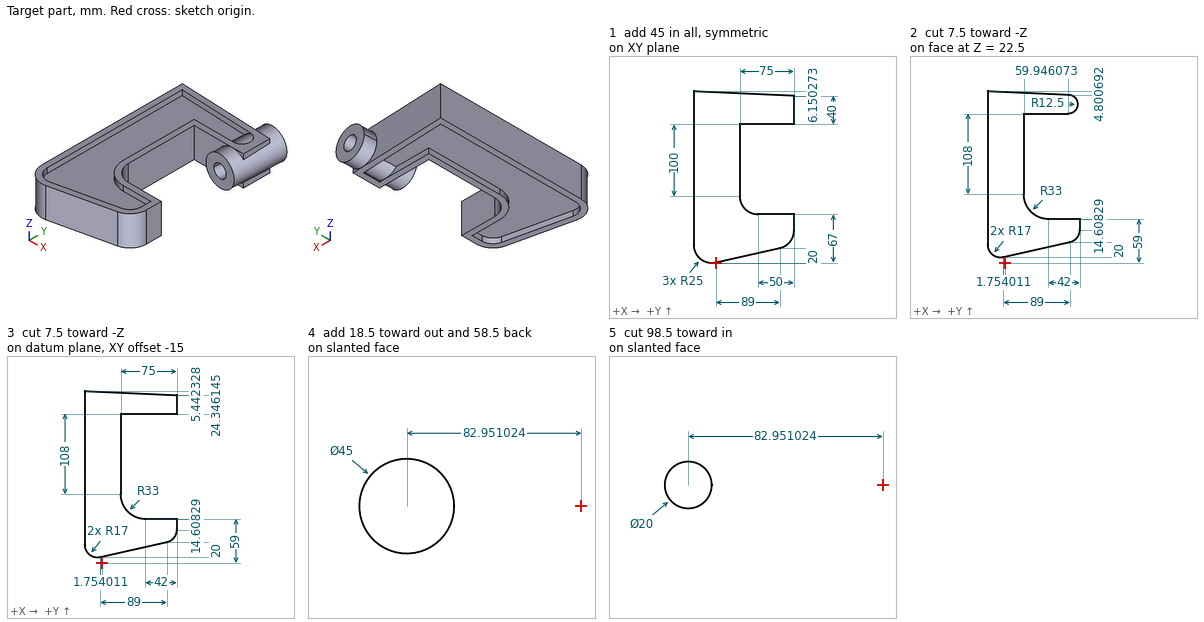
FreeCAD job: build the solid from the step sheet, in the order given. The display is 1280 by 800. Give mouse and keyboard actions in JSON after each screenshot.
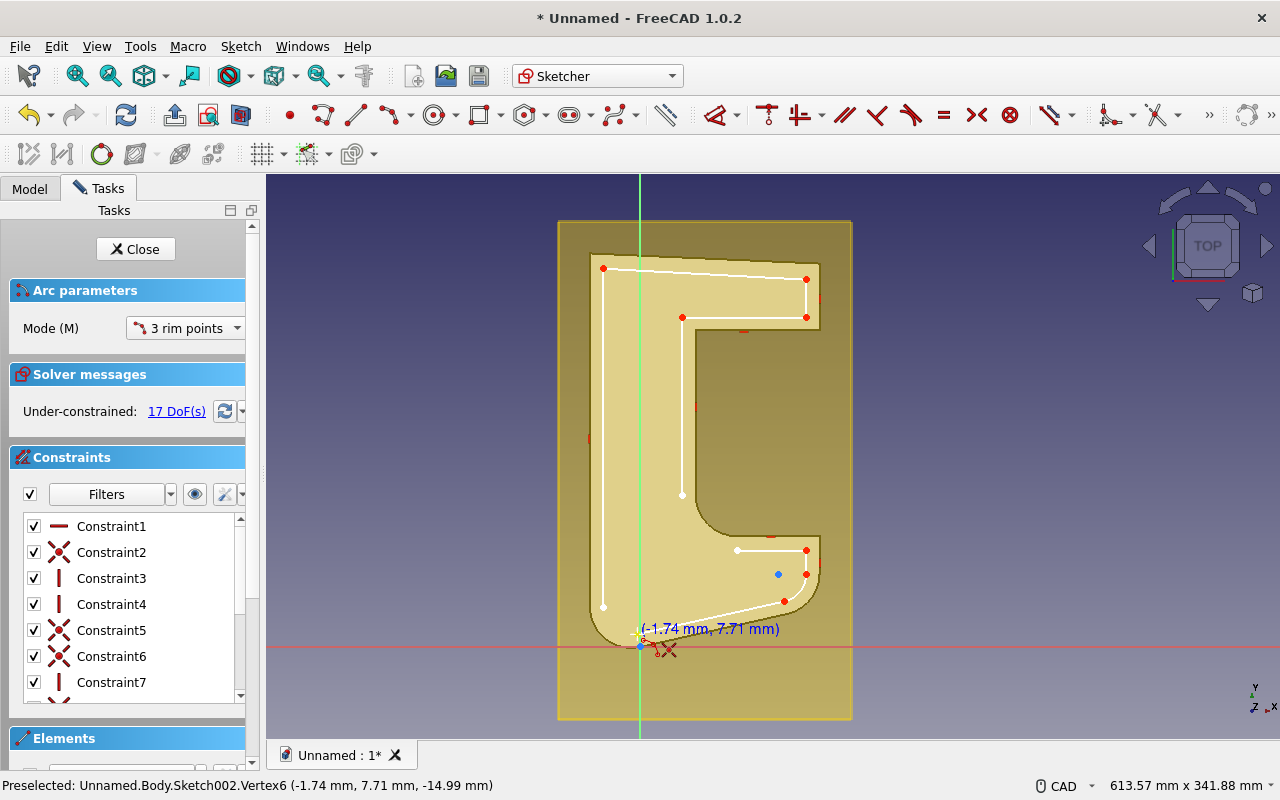
{"action": "left_click", "coordinate": [603, 608]}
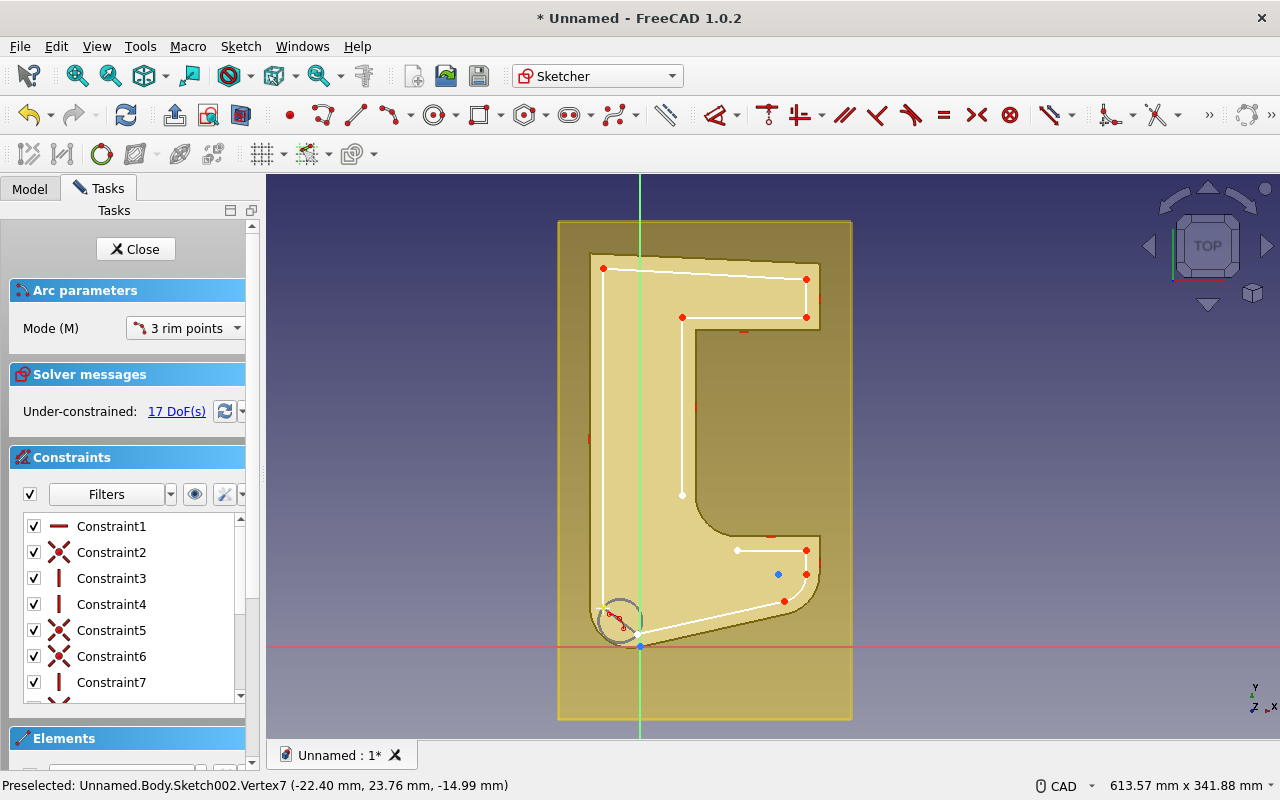
{"action": "scroll", "coordinate": [614, 629], "scroll_direction": "up", "scroll_amount": 3}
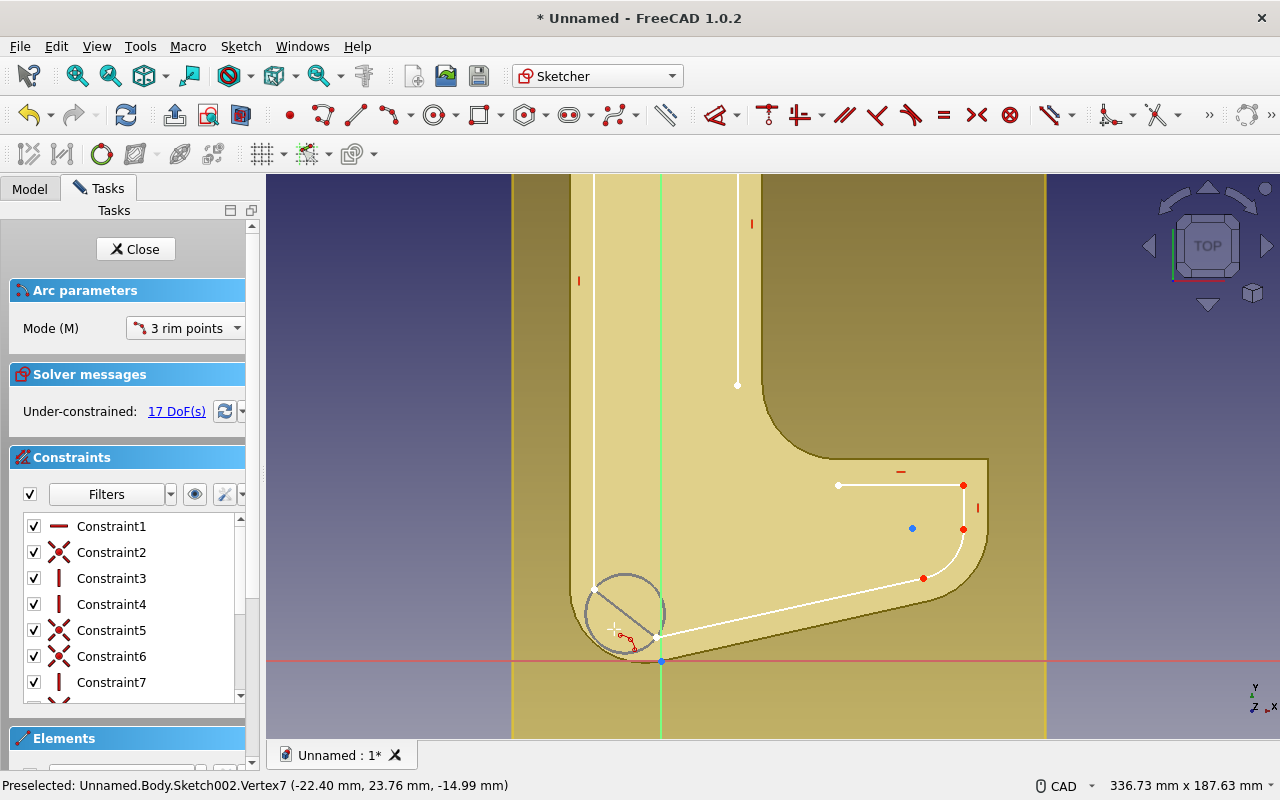
{"action": "left_click", "coordinate": [613, 628]}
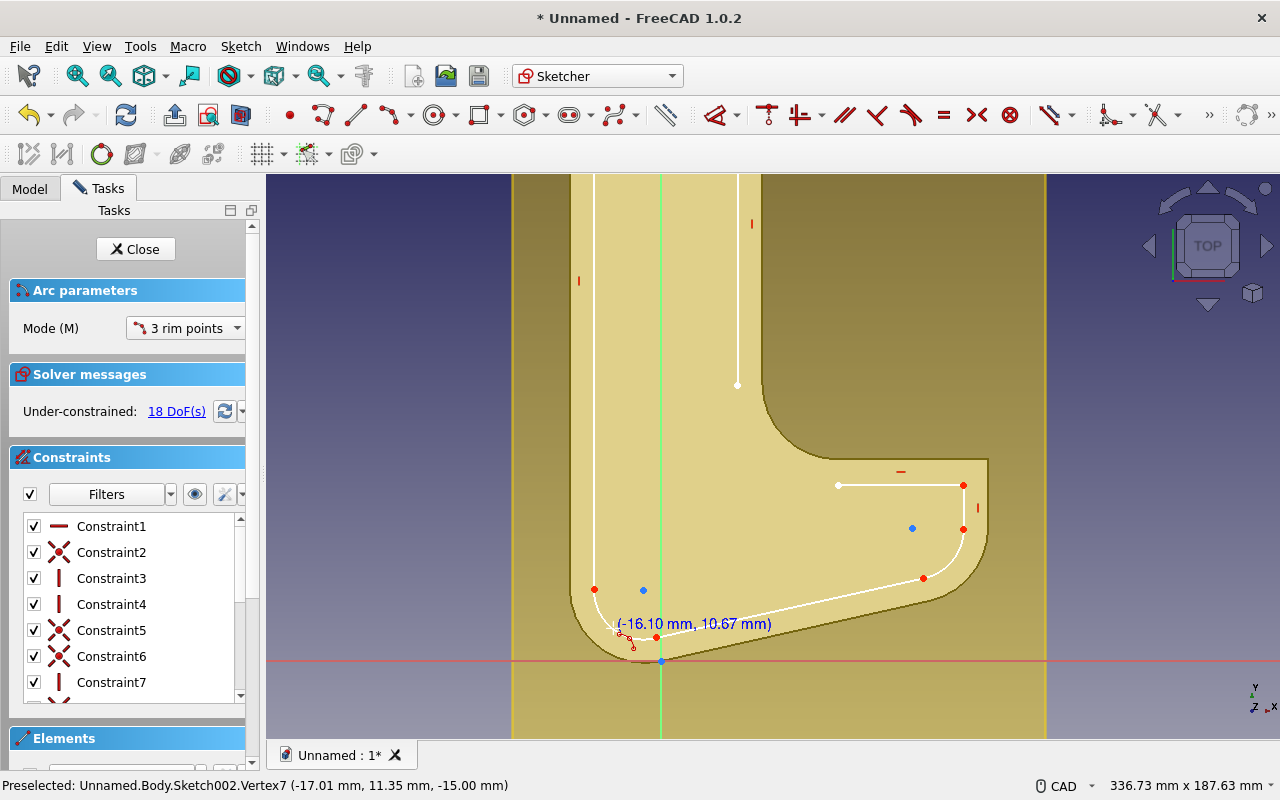
{"action": "left_click", "coordinate": [738, 385]}
{"action": "left_click", "coordinate": [838, 485]}
{"action": "left_click", "coordinate": [767, 454]}
{"action": "key", "text": "Escape"}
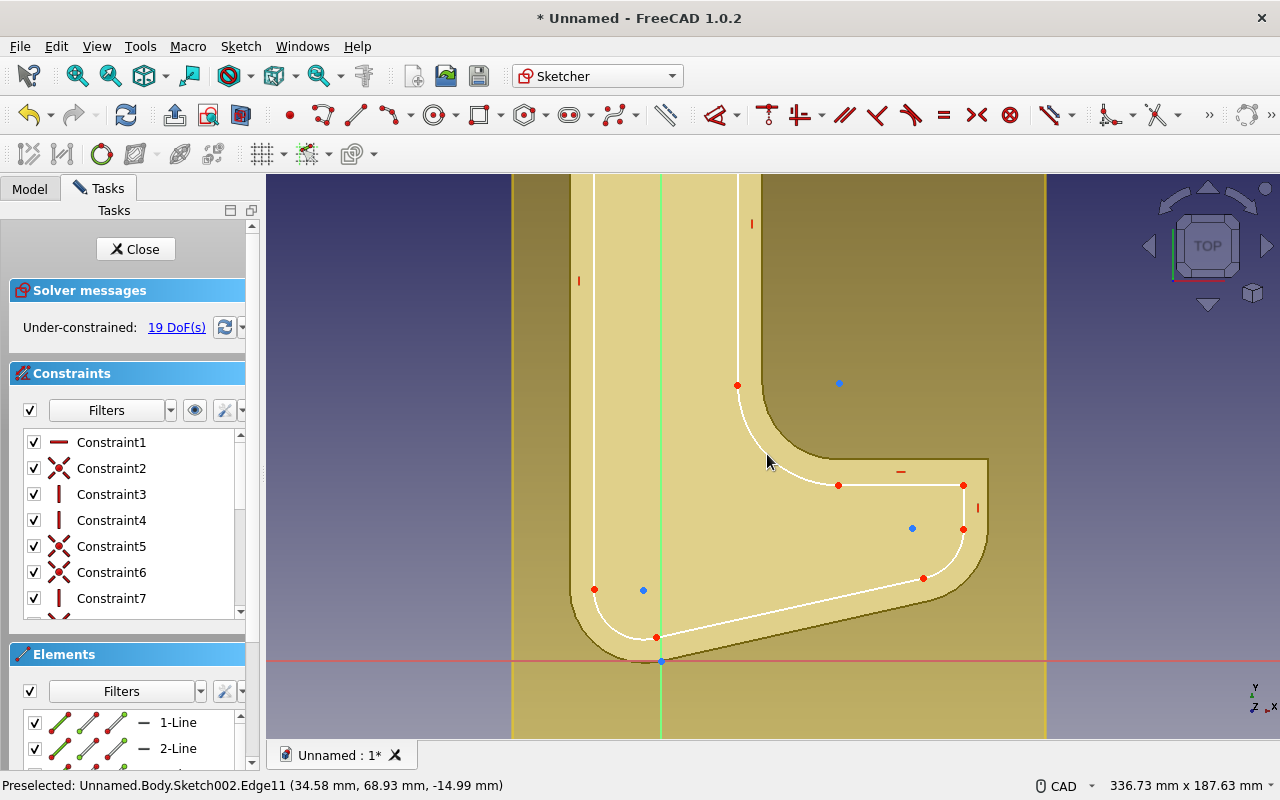
{"action": "left_click", "coordinate": [876, 485]}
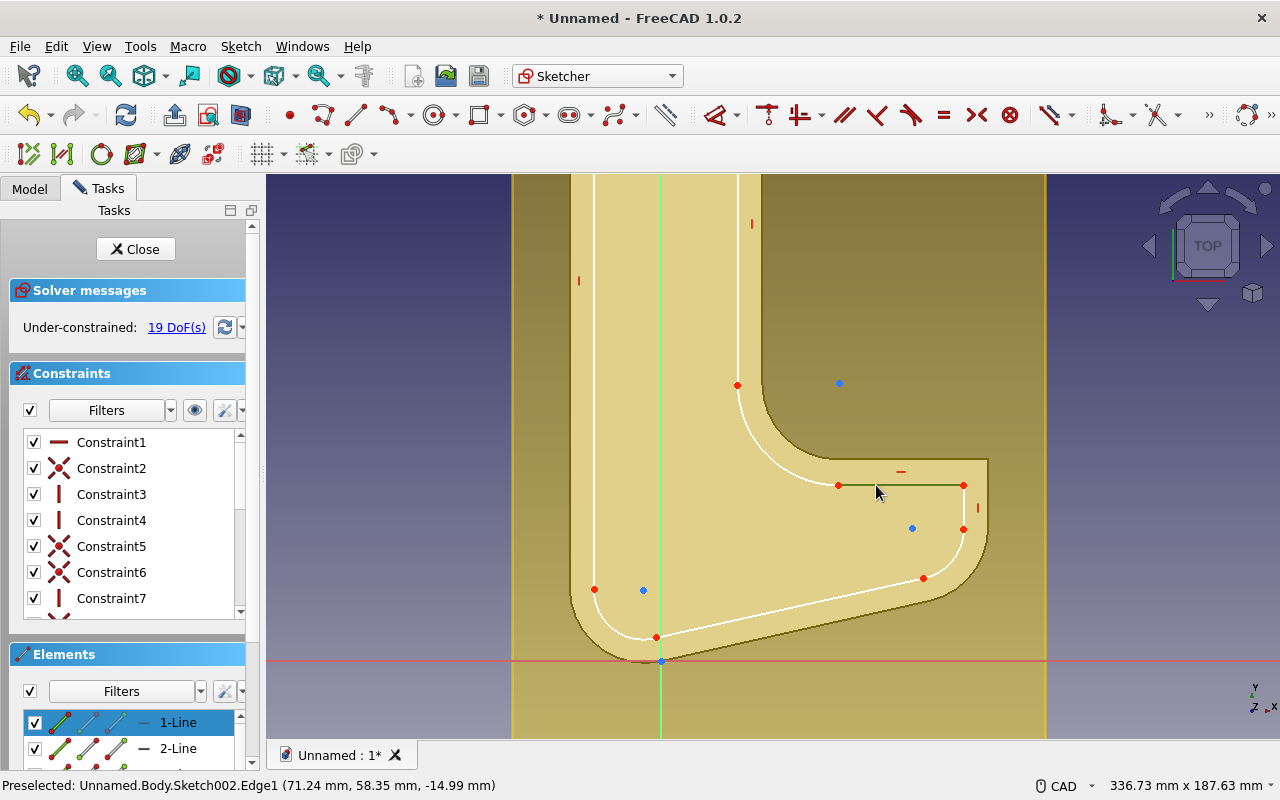
{"action": "left_click", "coordinate": [749, 431]}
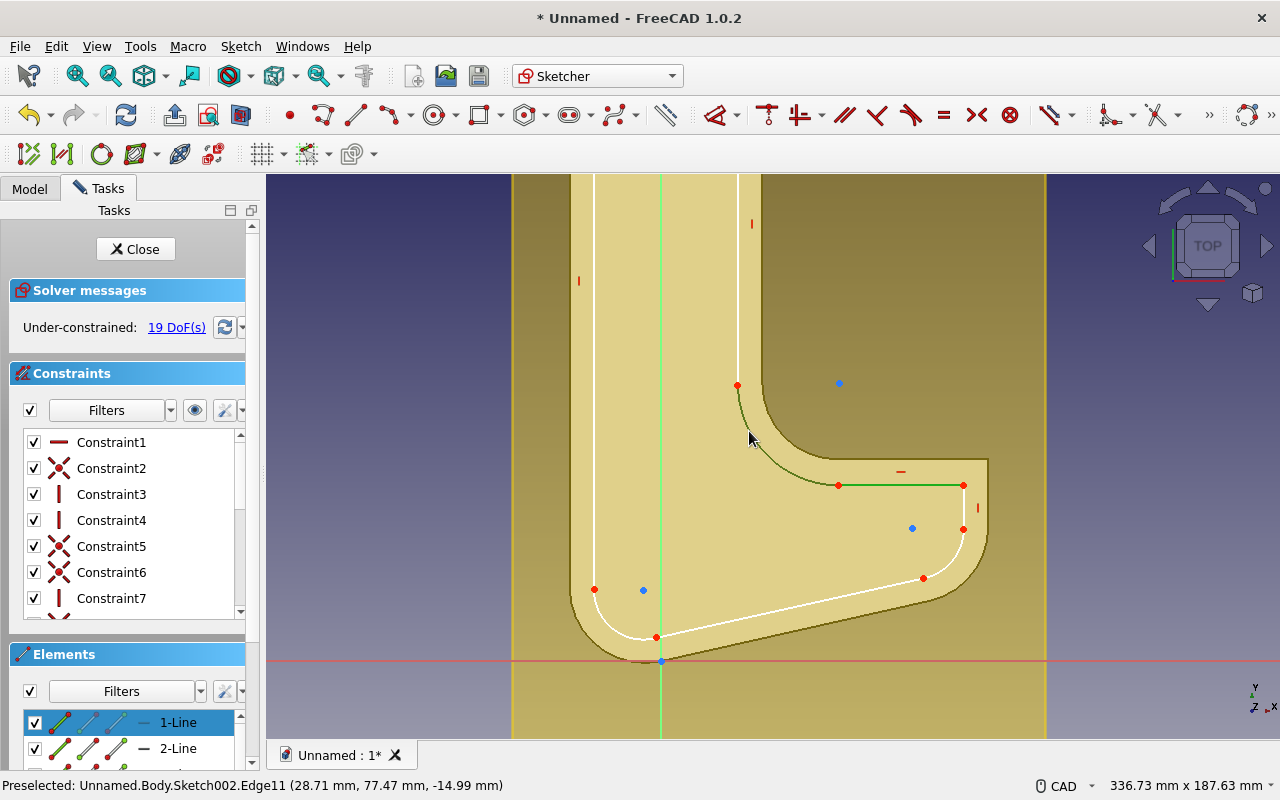
{"action": "left_click", "coordinate": [911, 116]}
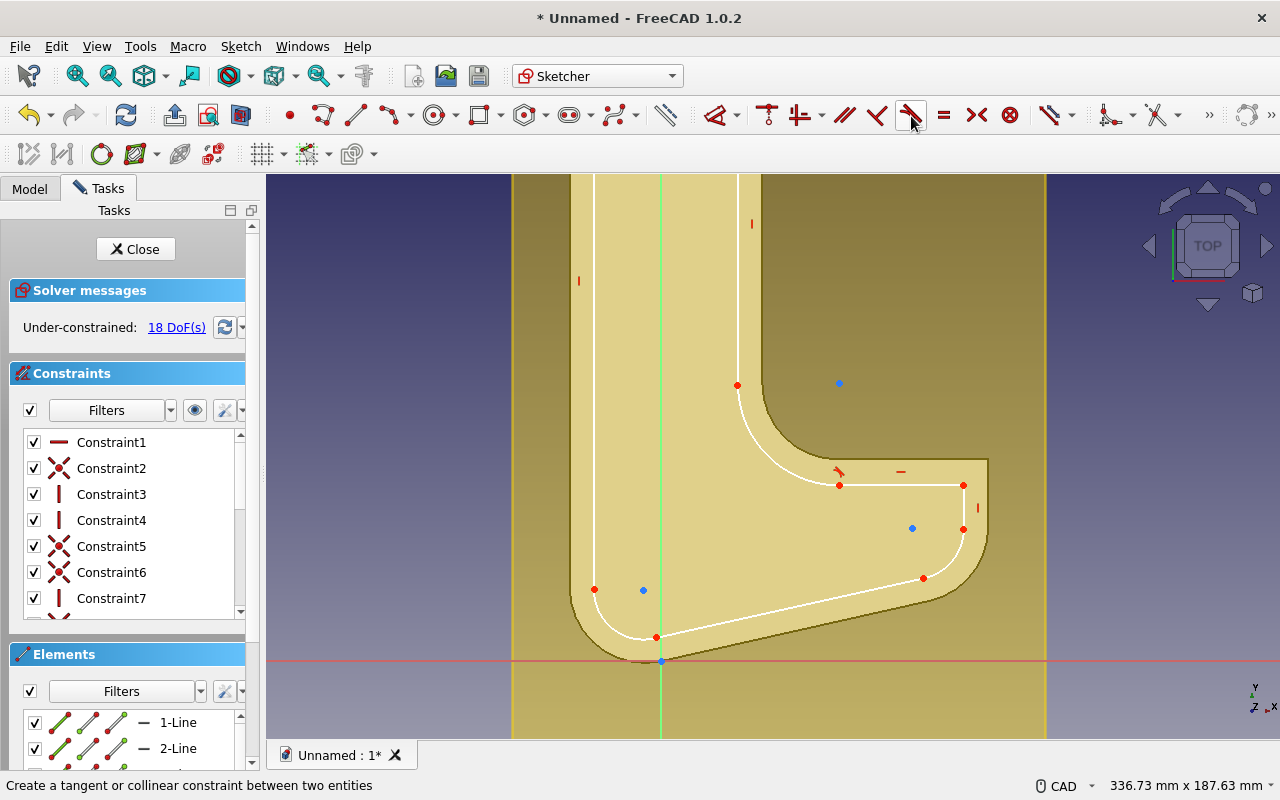
{"action": "left_click", "coordinate": [964, 499]}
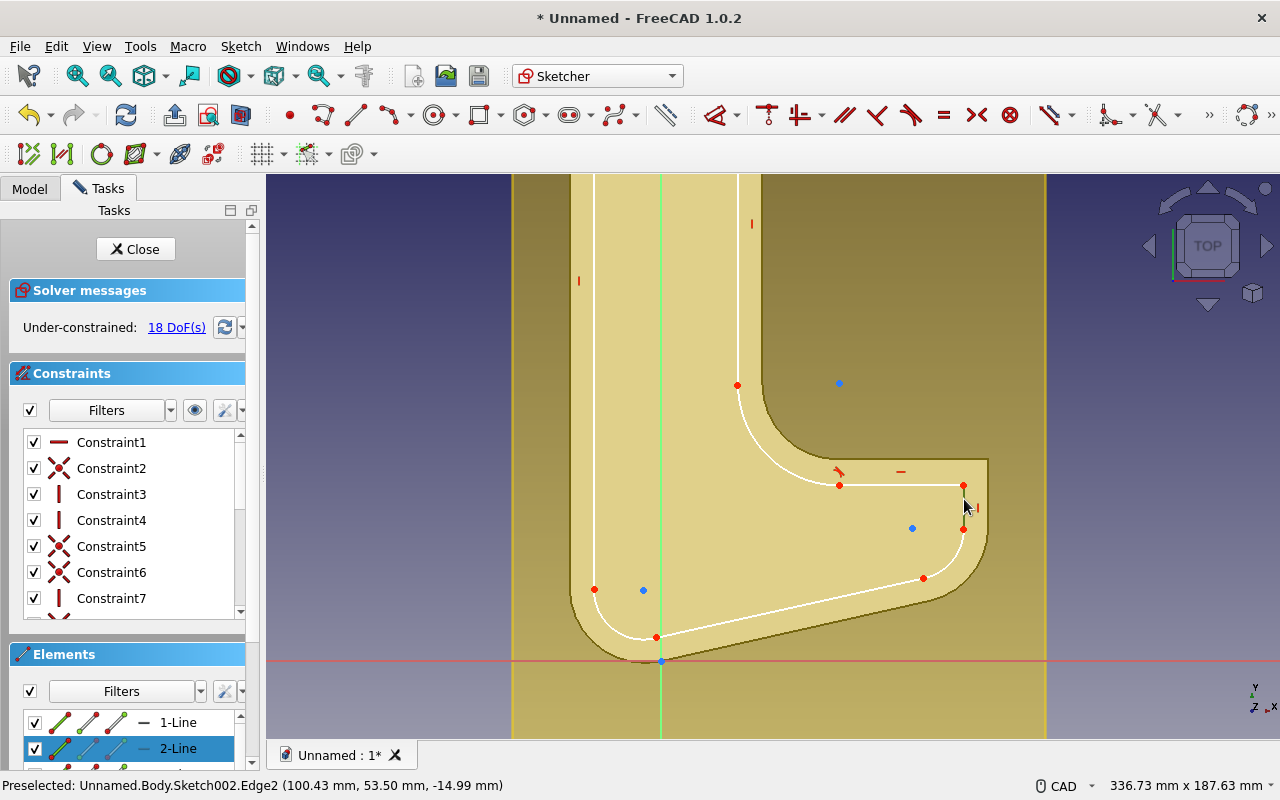
{"action": "left_click", "coordinate": [942, 570]}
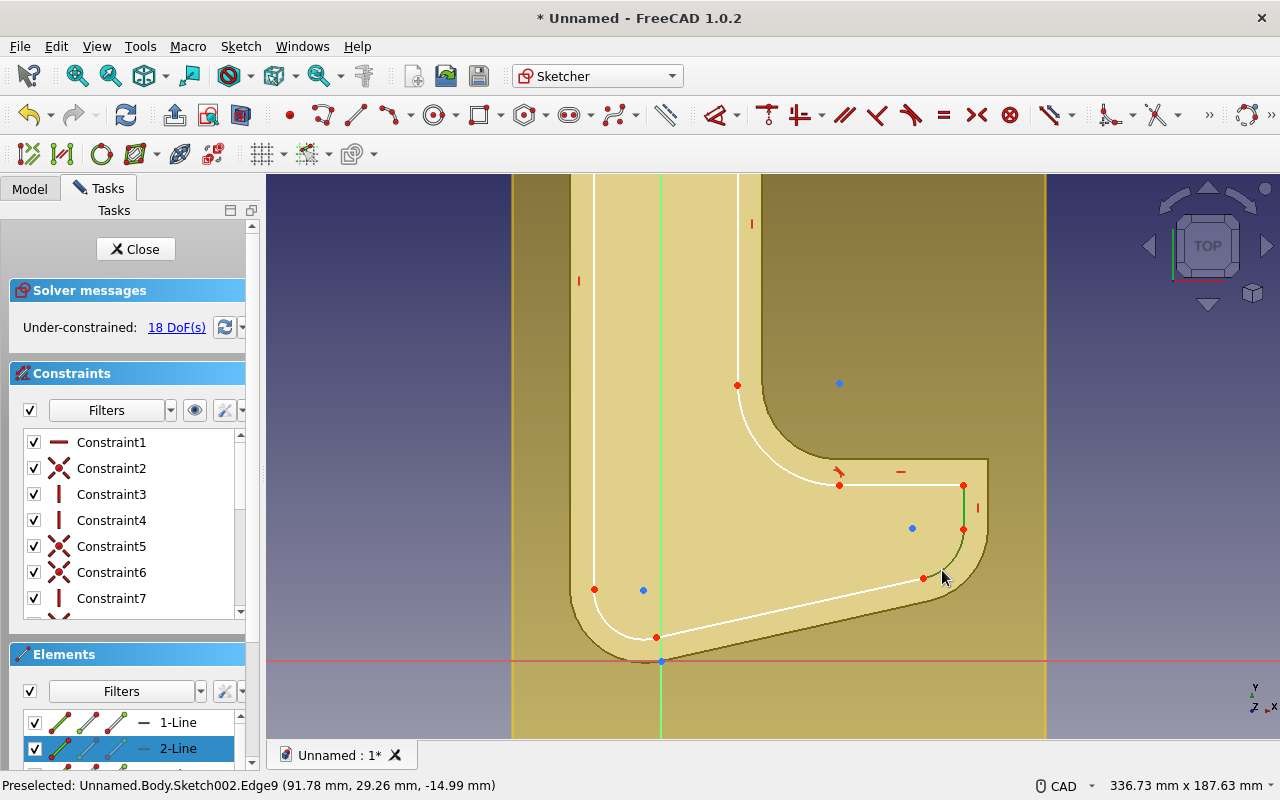
{"action": "left_click", "coordinate": [911, 116]}